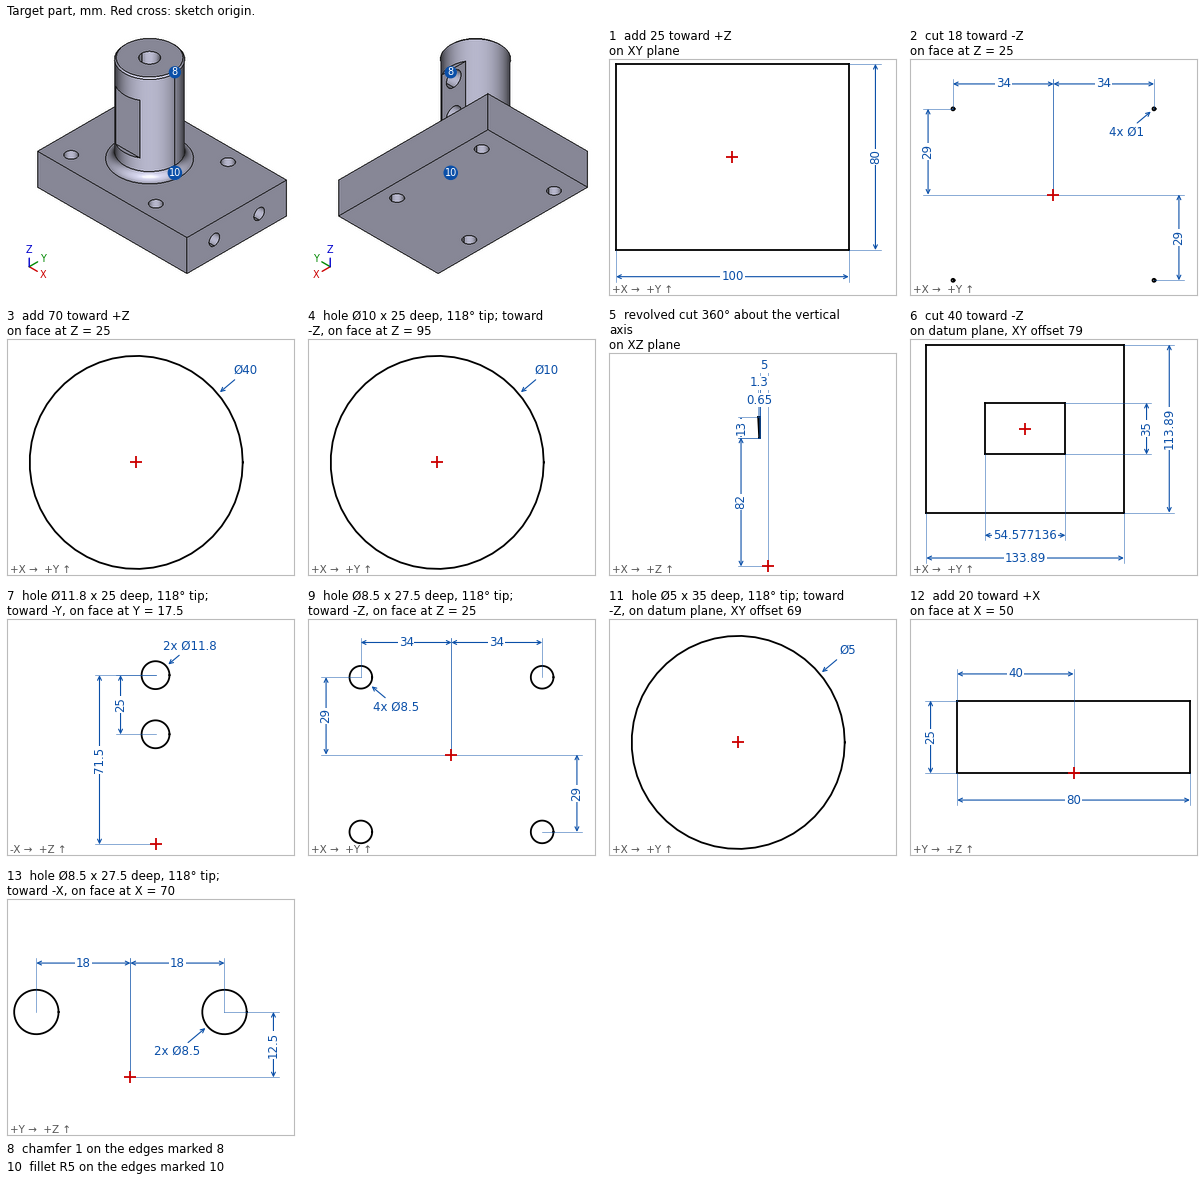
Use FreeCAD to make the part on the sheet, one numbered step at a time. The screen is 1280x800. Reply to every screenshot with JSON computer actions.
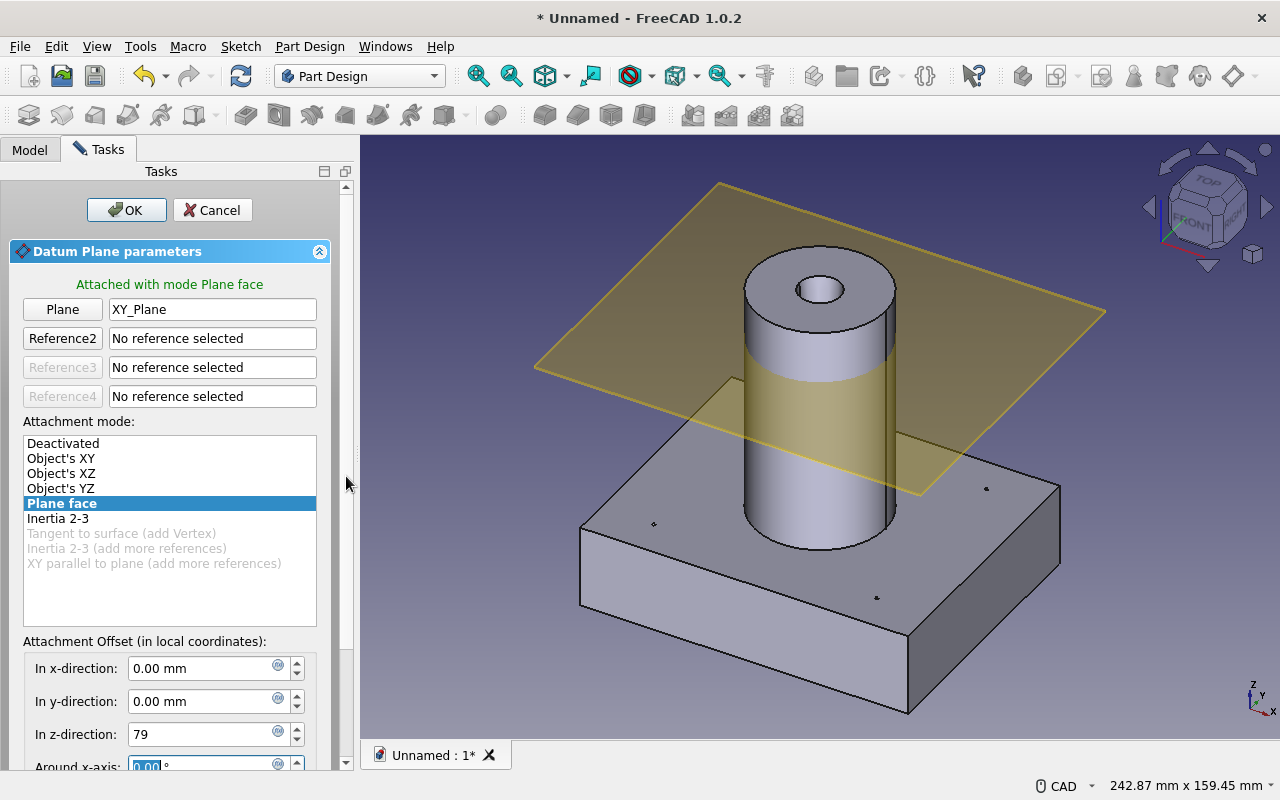
{"action": "left_click", "coordinate": [127, 210]}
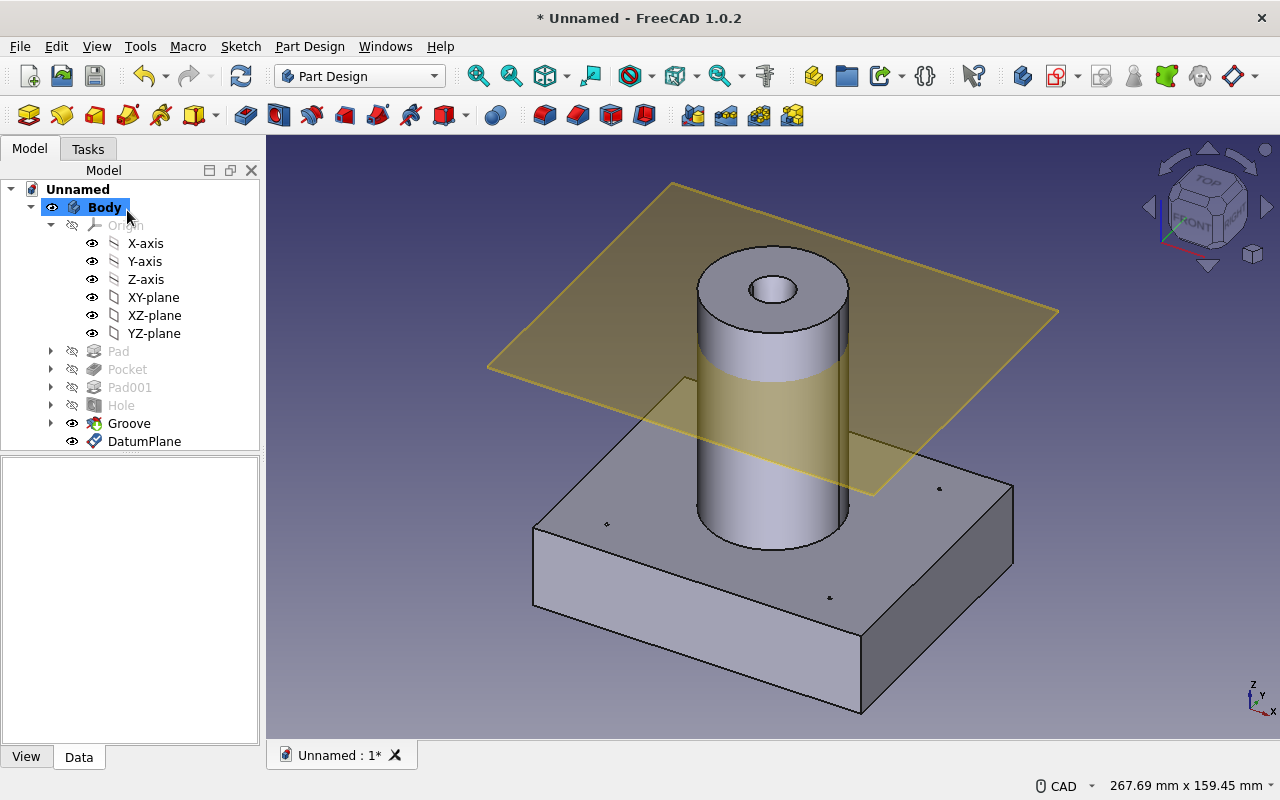
{"action": "left_click", "coordinate": [117, 441]}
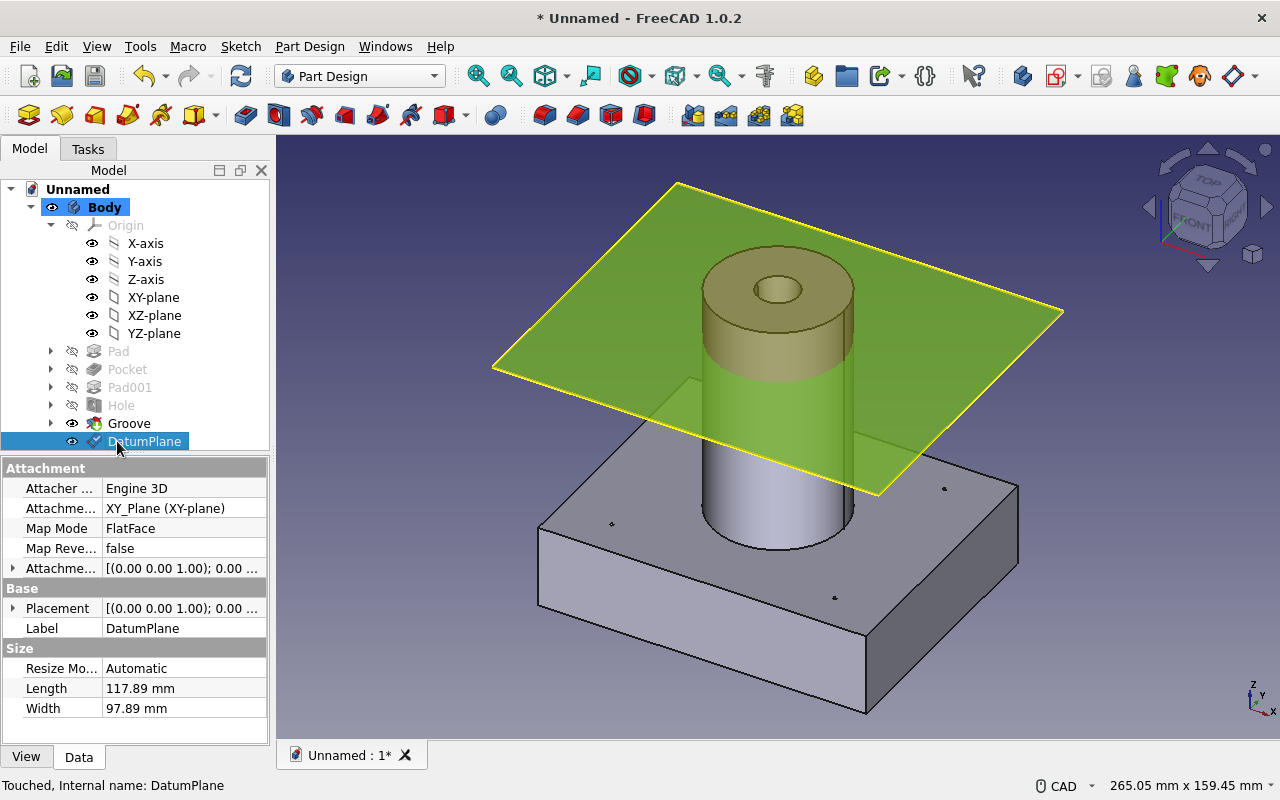
{"action": "left_click", "coordinate": [1056, 76]}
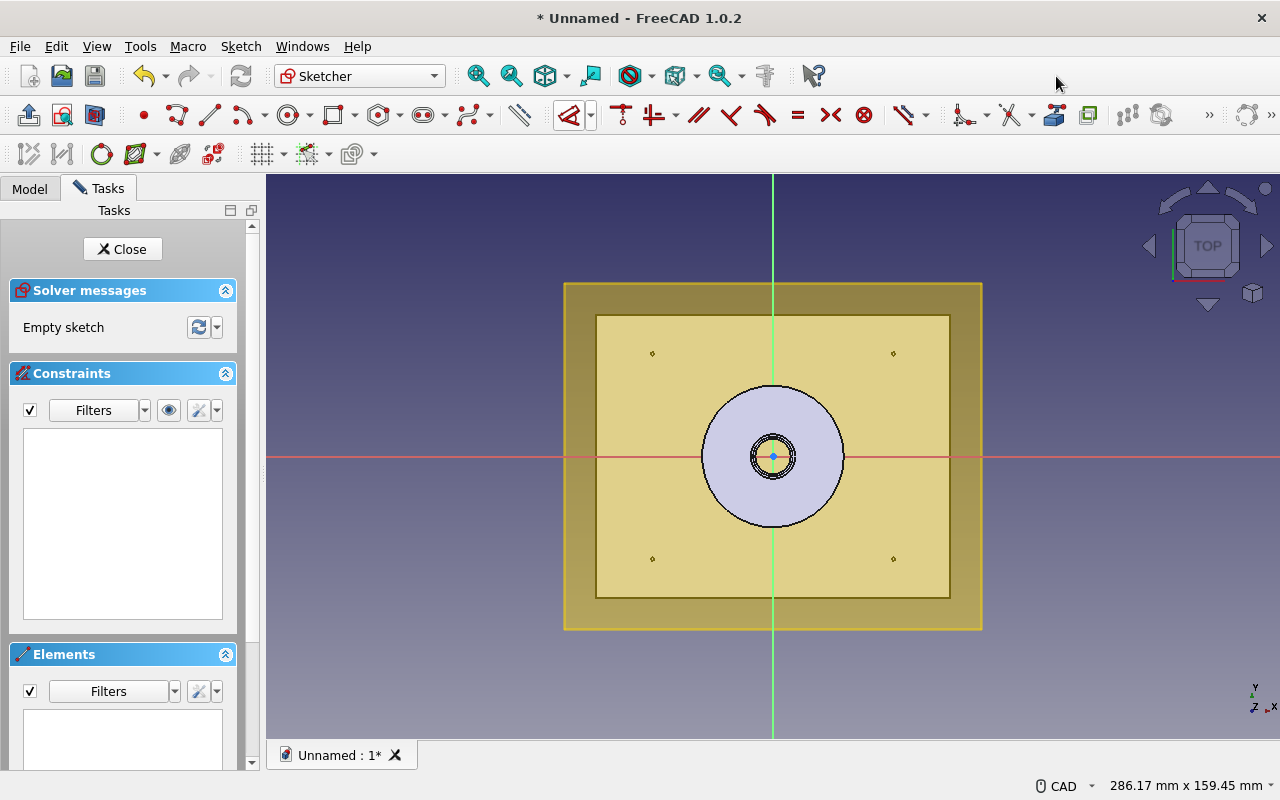
{"action": "left_click", "coordinate": [95, 116]}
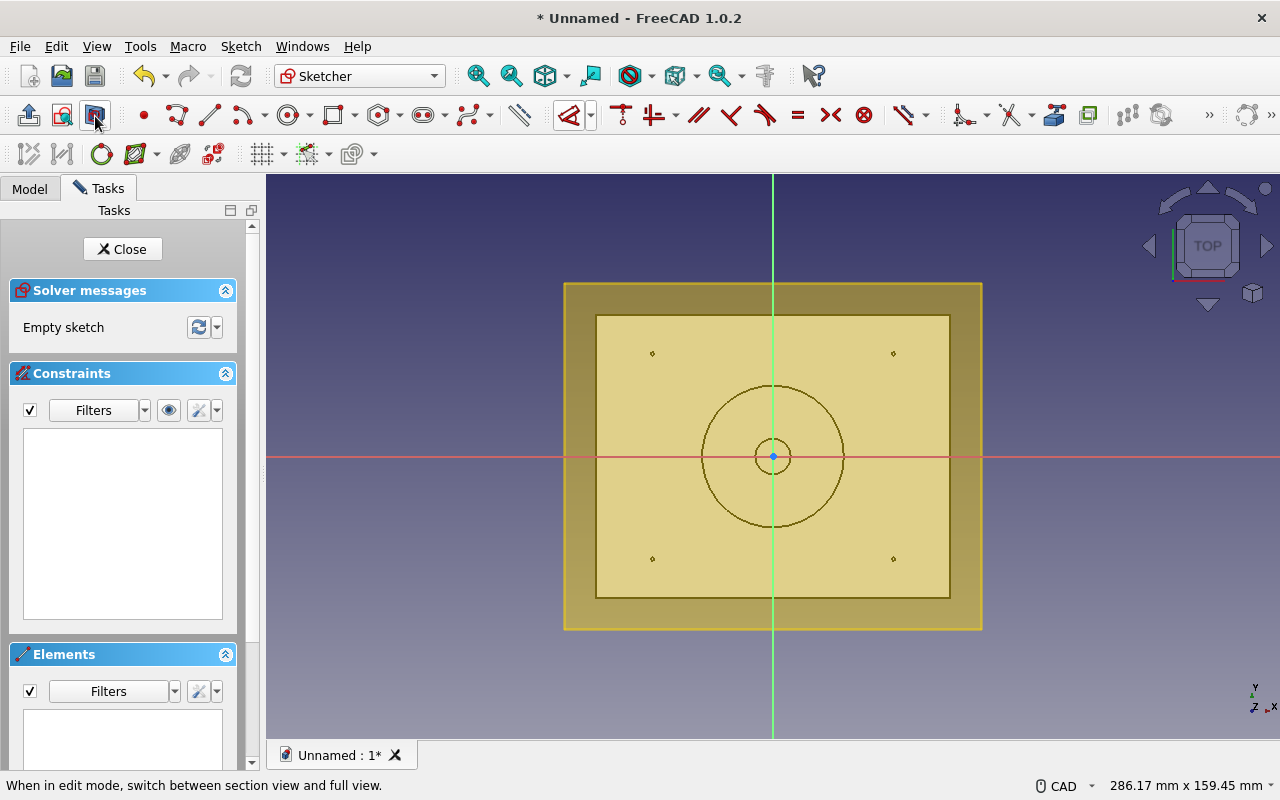
{"action": "key", "text": "g v"}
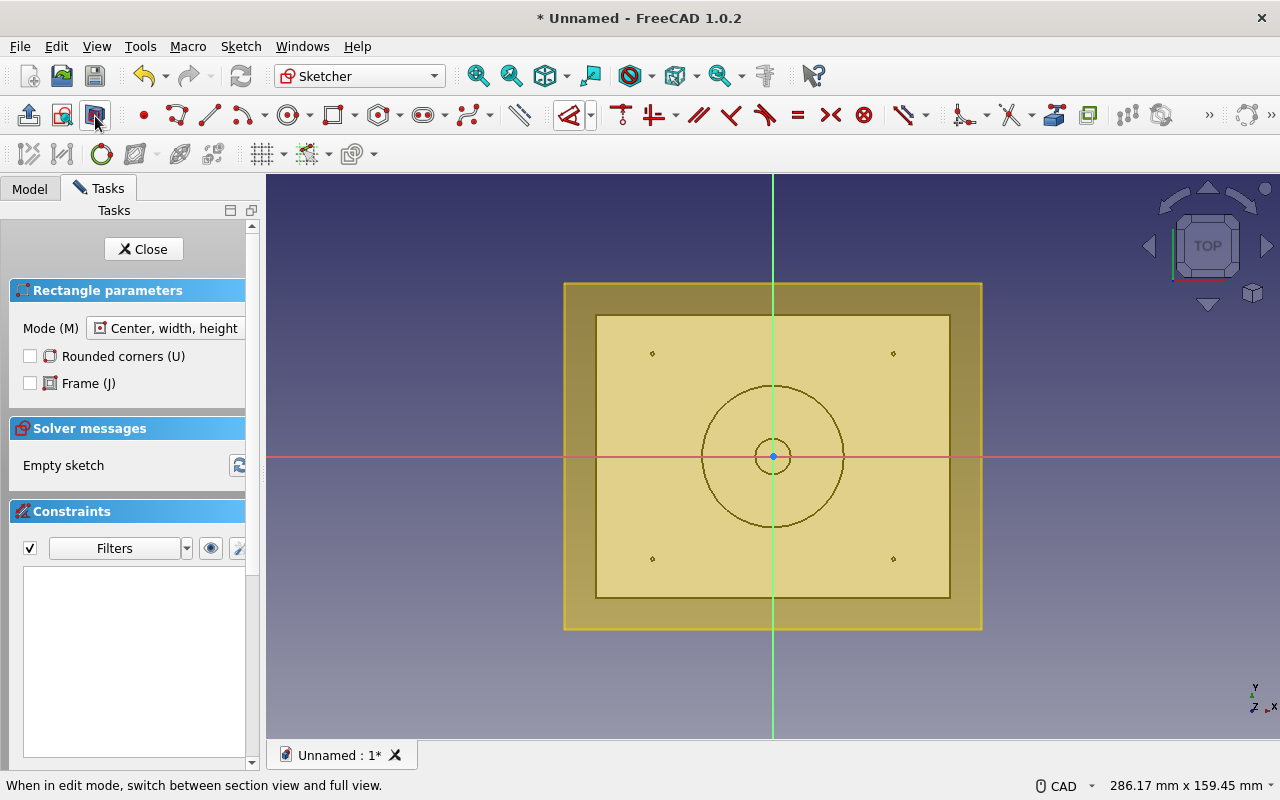
{"action": "left_click", "coordinate": [773, 456]}
{"action": "mouse_move", "coordinate": [1010, 255]}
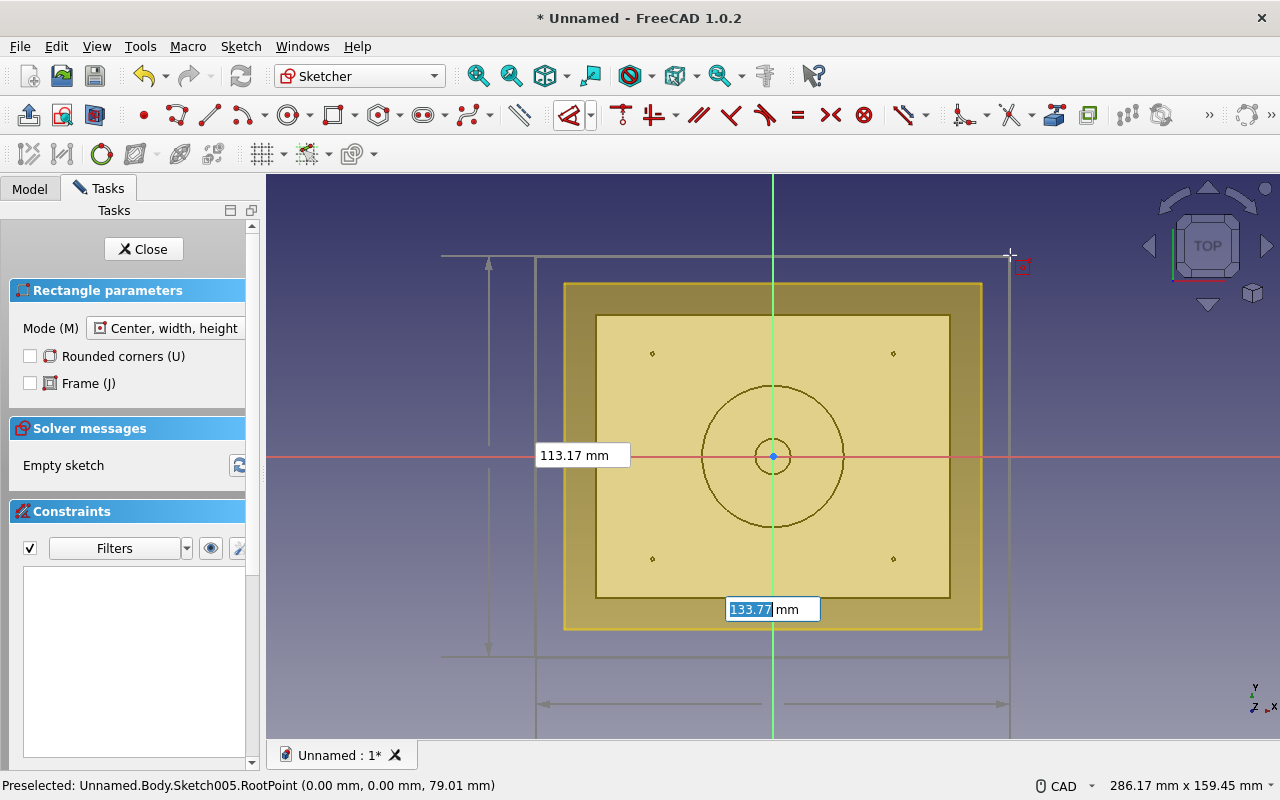
{"action": "type", "text": "133.89"}
{"action": "key", "text": "Tab"}
{"action": "type", "text": "113.89"}
{"action": "key", "text": "Return"}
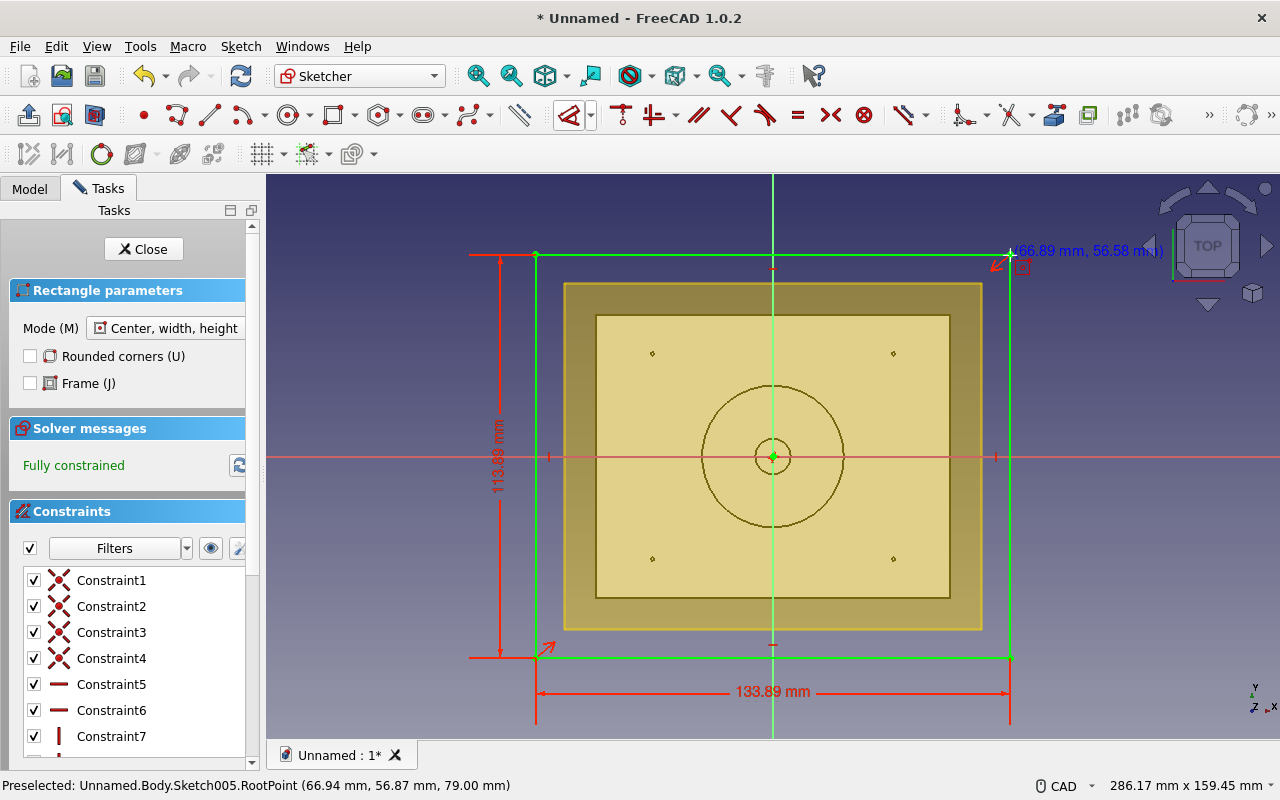
{"action": "left_click", "coordinate": [773, 456]}
{"action": "mouse_move", "coordinate": [870, 394]}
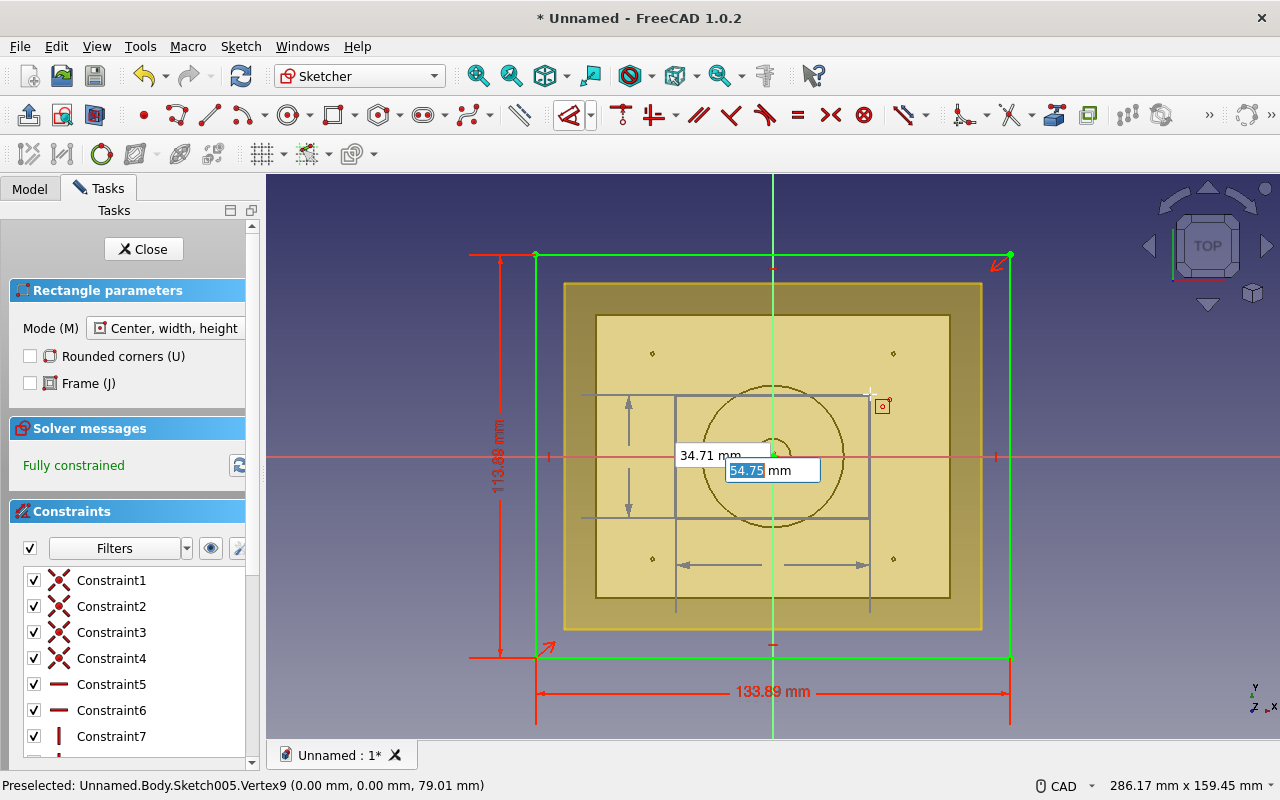
{"action": "type", "text": "54.577136"}
{"action": "key", "text": "Tab"}
{"action": "type", "text": "35"}
{"action": "key", "text": "Return"}
{"action": "key", "text": "Escape"}